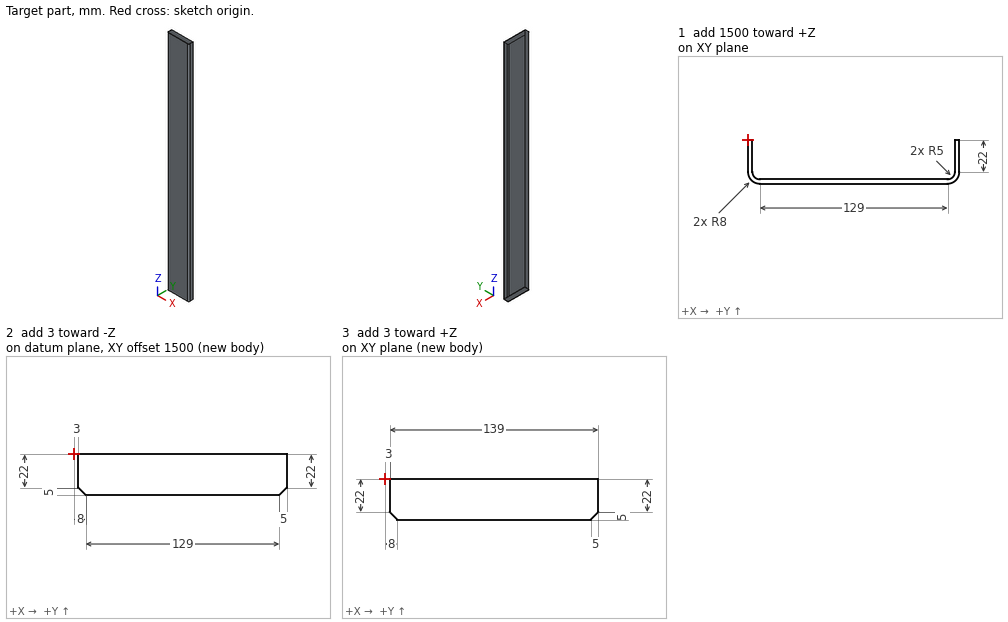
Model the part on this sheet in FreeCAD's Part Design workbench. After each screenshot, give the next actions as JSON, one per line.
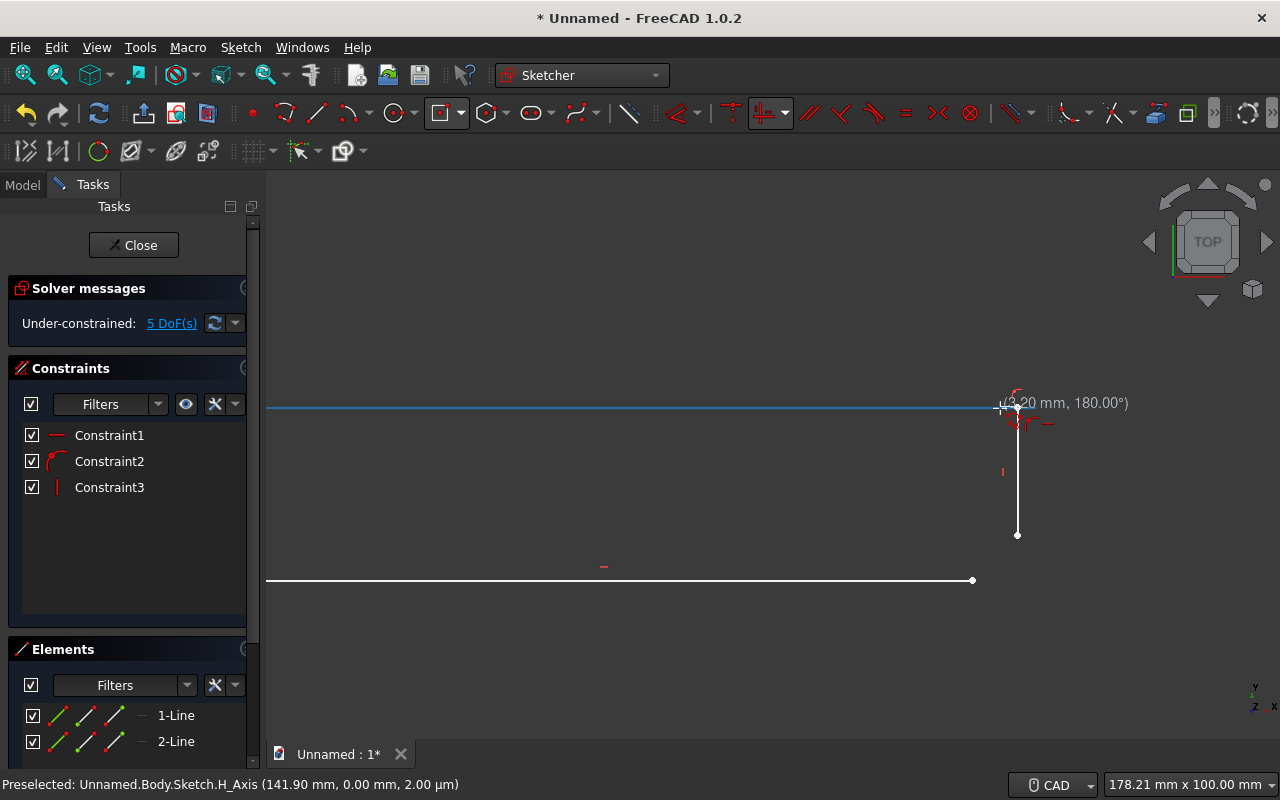
{"action": "left_click", "coordinate": [1000, 417]}
{"action": "left_click", "coordinate": [1000, 533]}
{"action": "right_click", "coordinate": [1000, 533]}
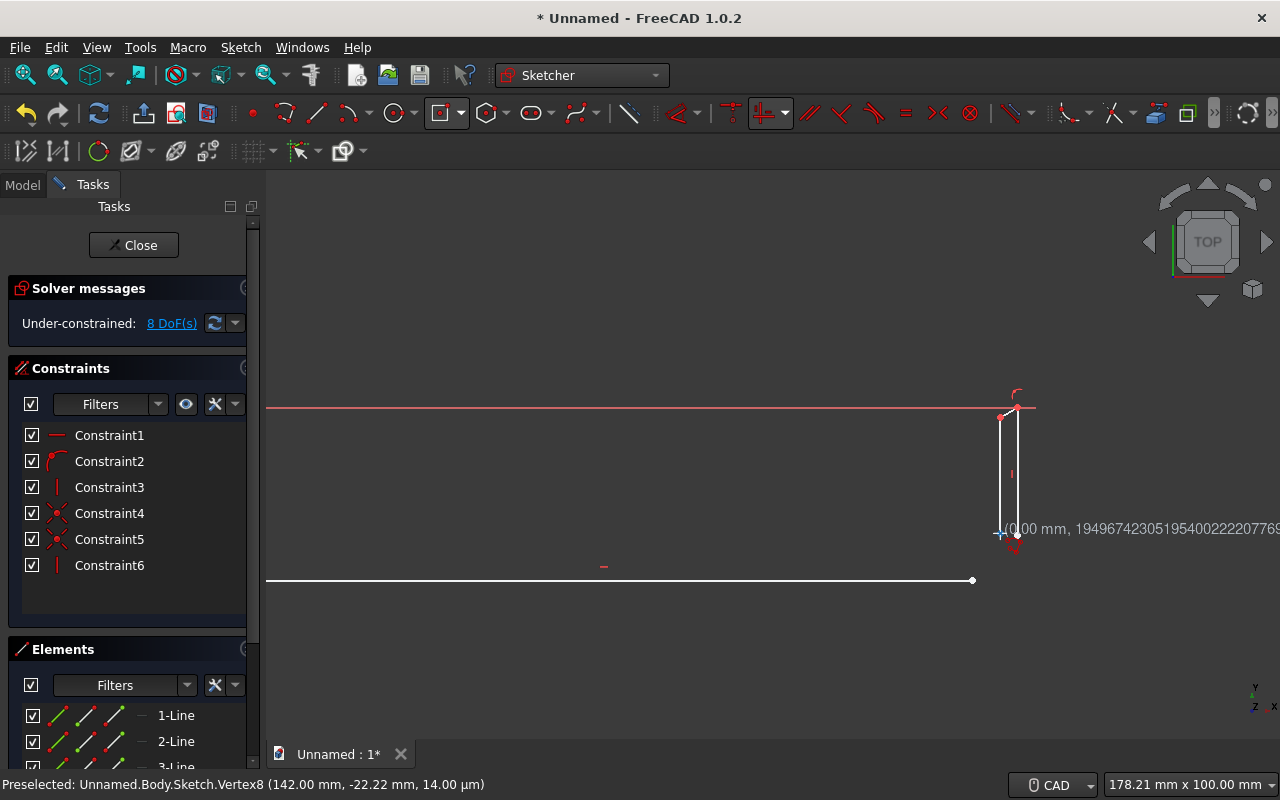
{"action": "key", "text": "g l"}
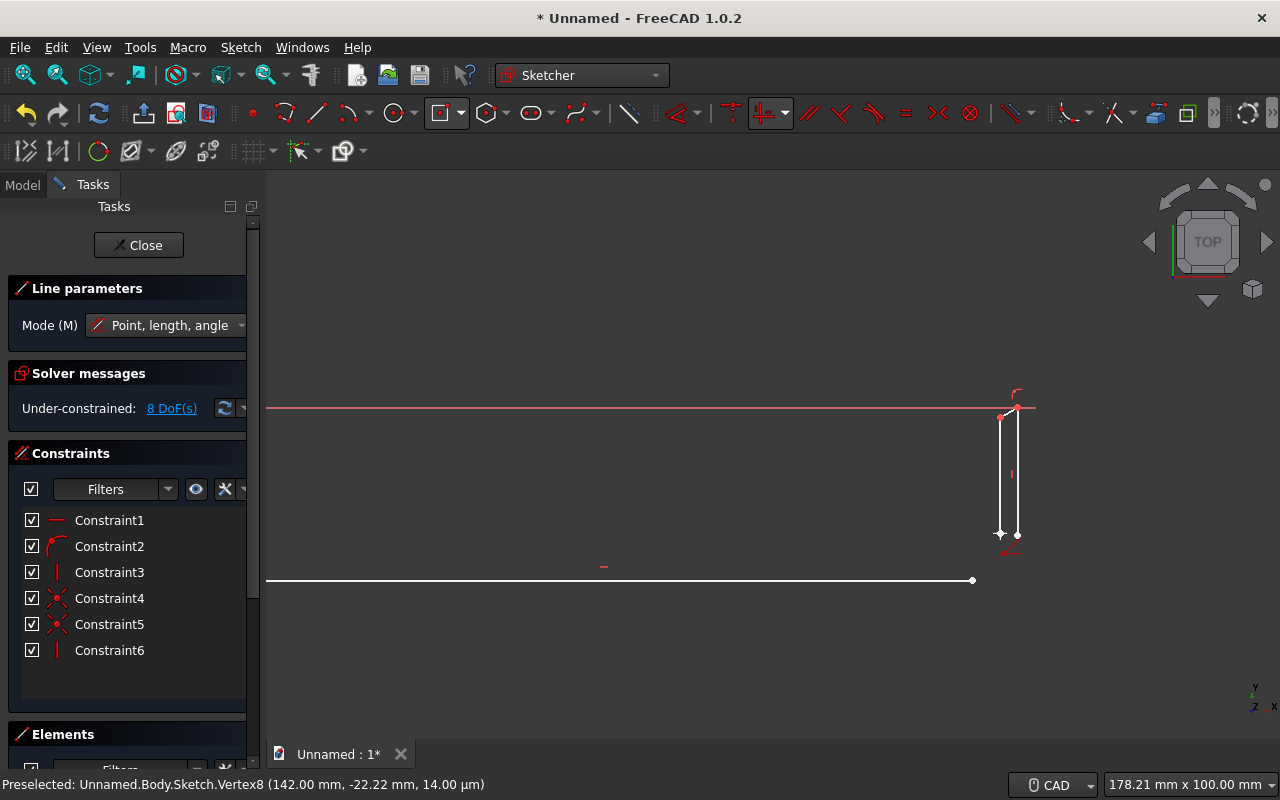
{"action": "left_click", "coordinate": [972, 561]}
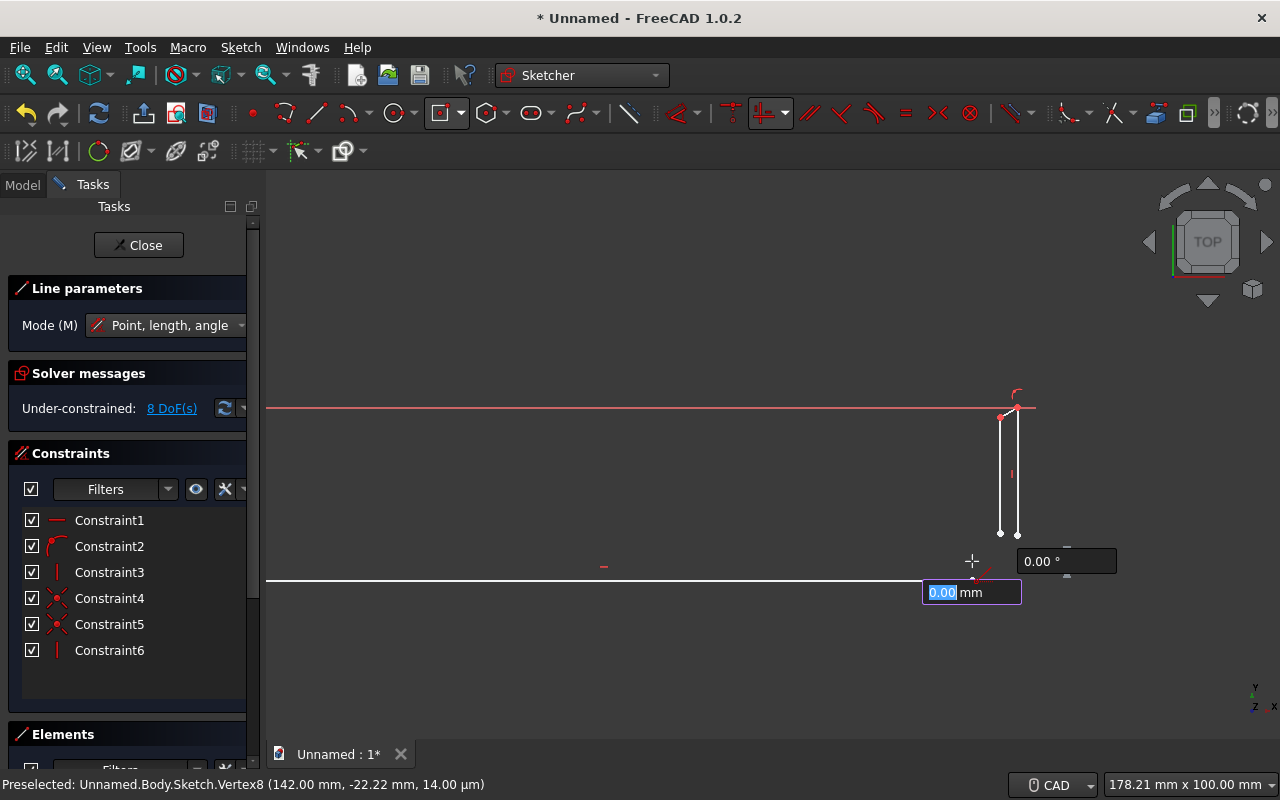
{"action": "scroll", "coordinate": [908, 376], "scroll_direction": "down", "scroll_amount": 2}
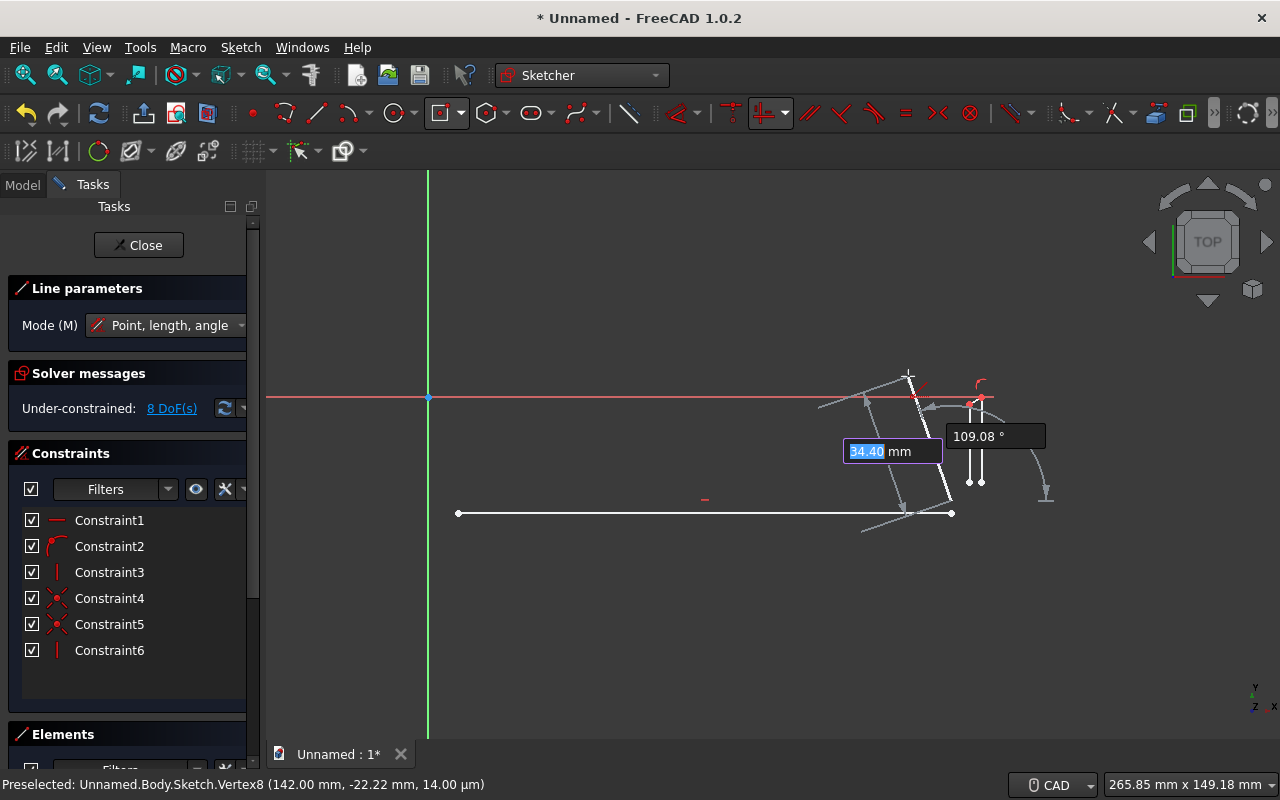
{"action": "scroll", "coordinate": [459, 500], "scroll_direction": "up", "scroll_amount": 2}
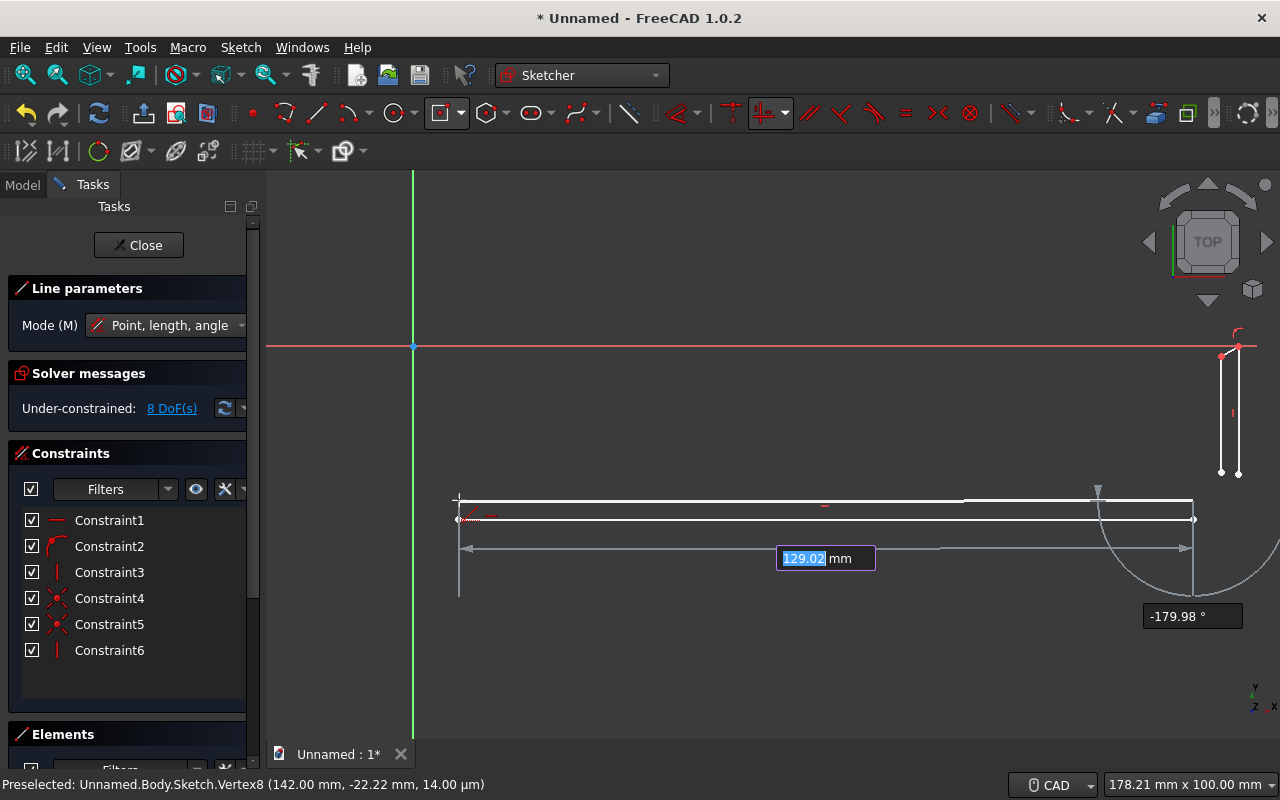
{"action": "left_click", "coordinate": [459, 500]}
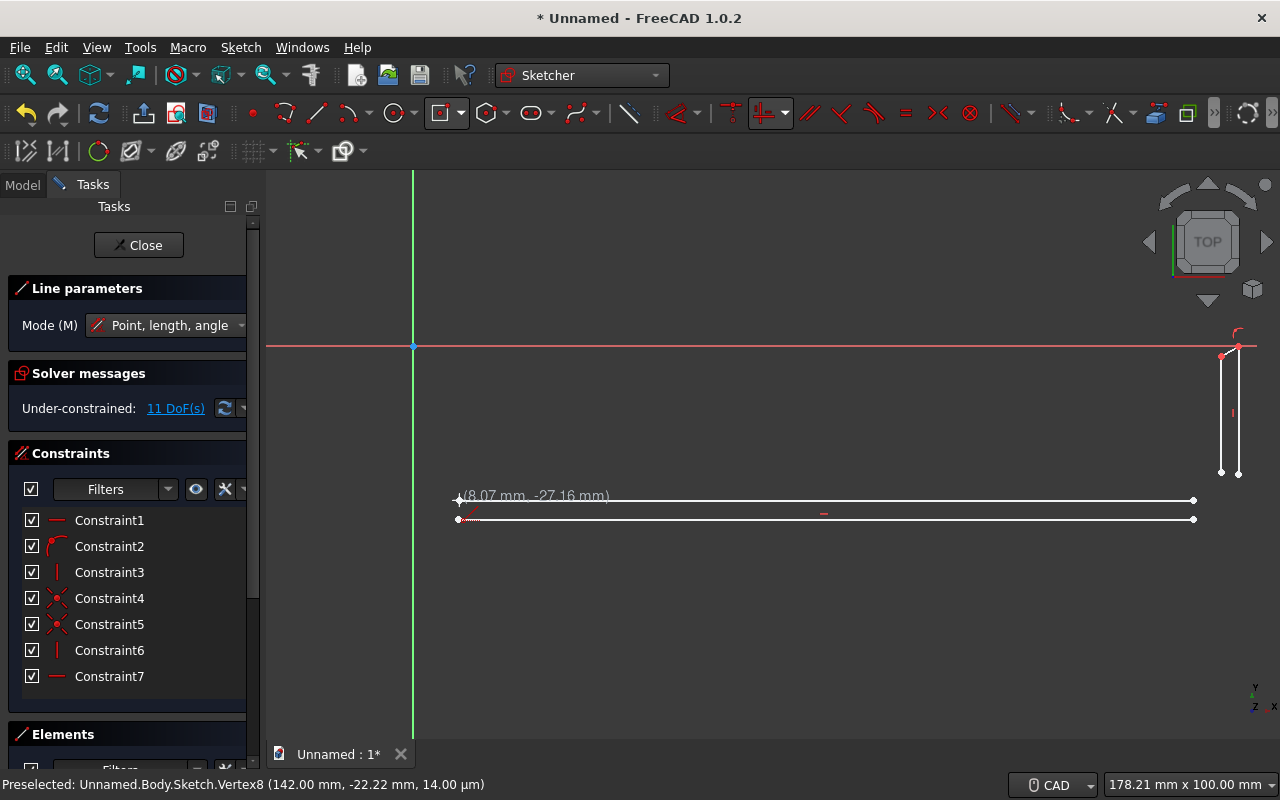
{"action": "key", "text": "g m"}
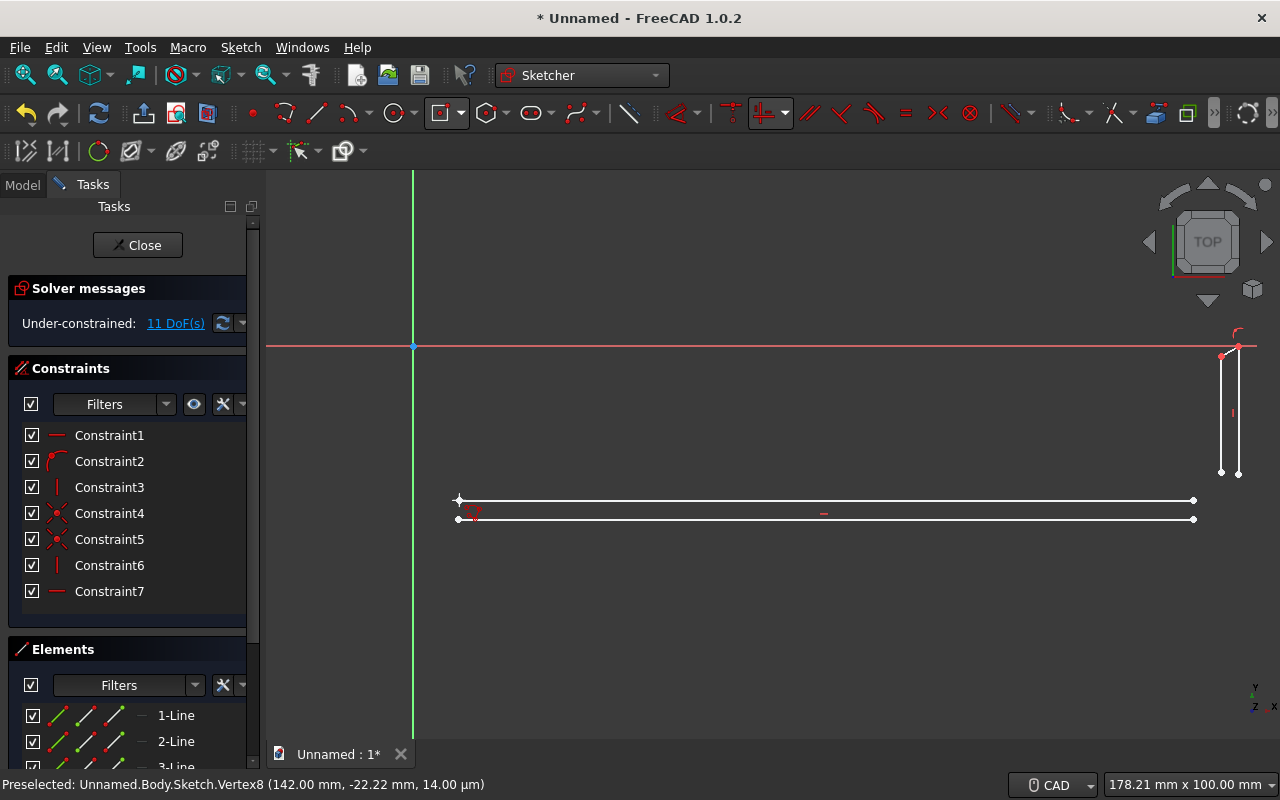
{"action": "left_click", "coordinate": [430, 472]}
{"action": "left_click", "coordinate": [430, 346]}
{"action": "left_click", "coordinate": [413, 346]}
{"action": "left_click", "coordinate": [422, 472]}
{"action": "right_click", "coordinate": [422, 472]}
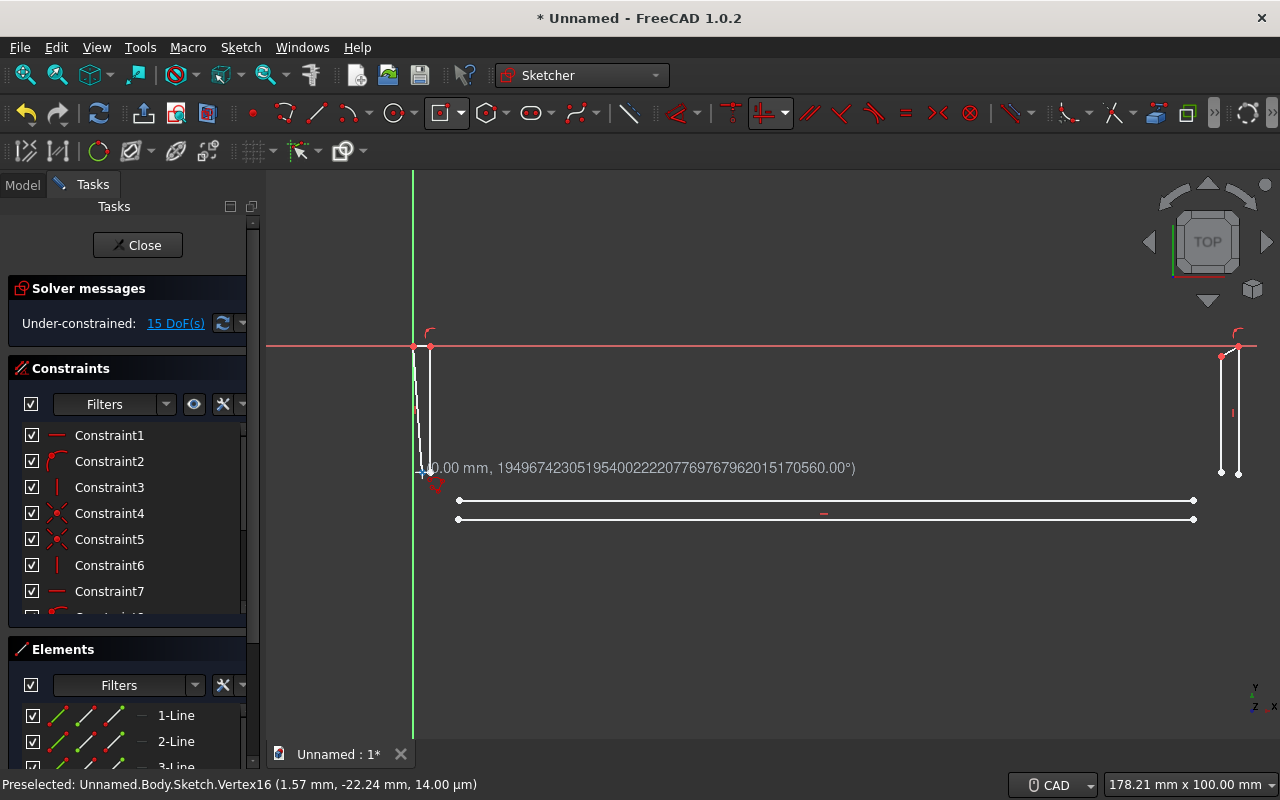
{"action": "key", "text": "g 3 a"}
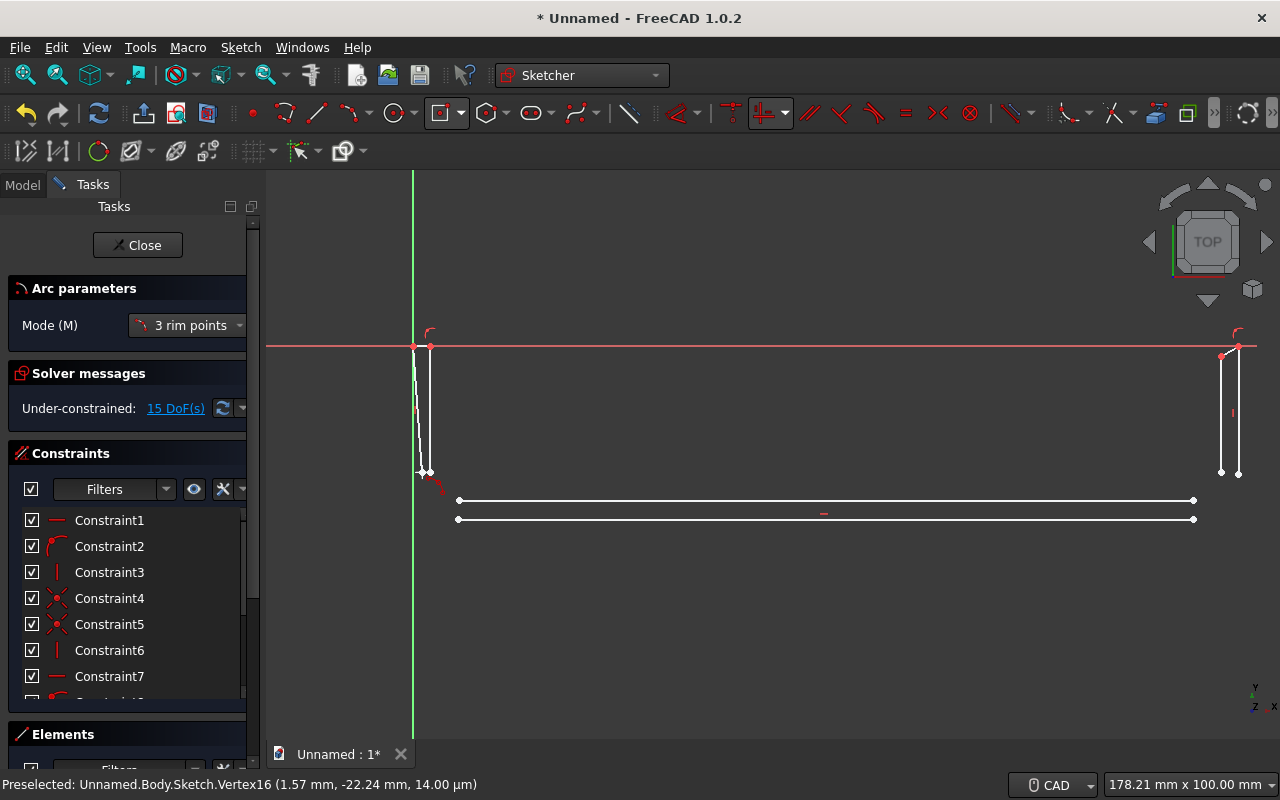
{"action": "scroll", "coordinate": [458, 501], "scroll_direction": "down", "scroll_amount": 2}